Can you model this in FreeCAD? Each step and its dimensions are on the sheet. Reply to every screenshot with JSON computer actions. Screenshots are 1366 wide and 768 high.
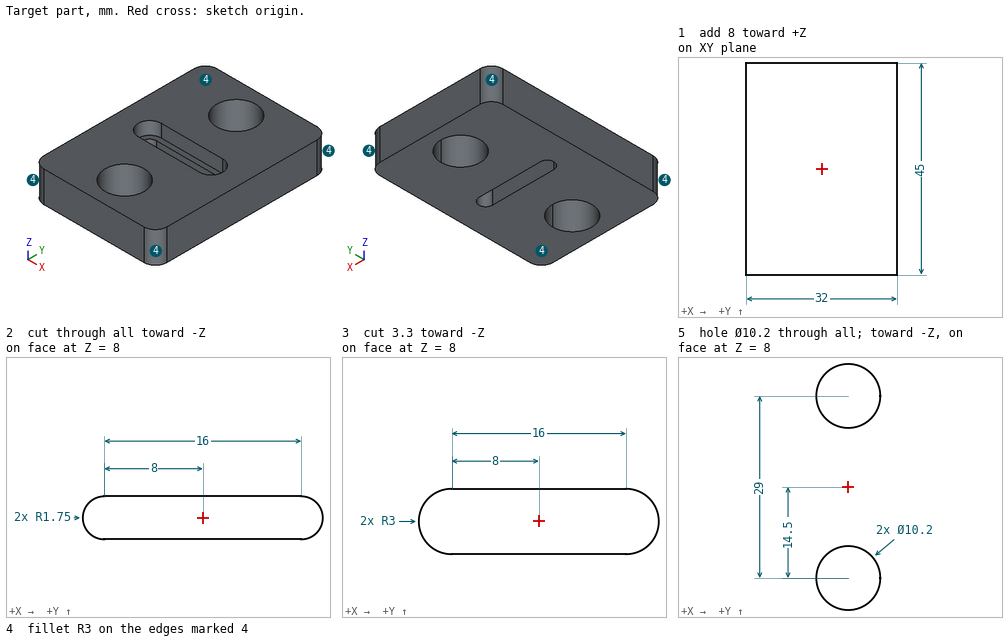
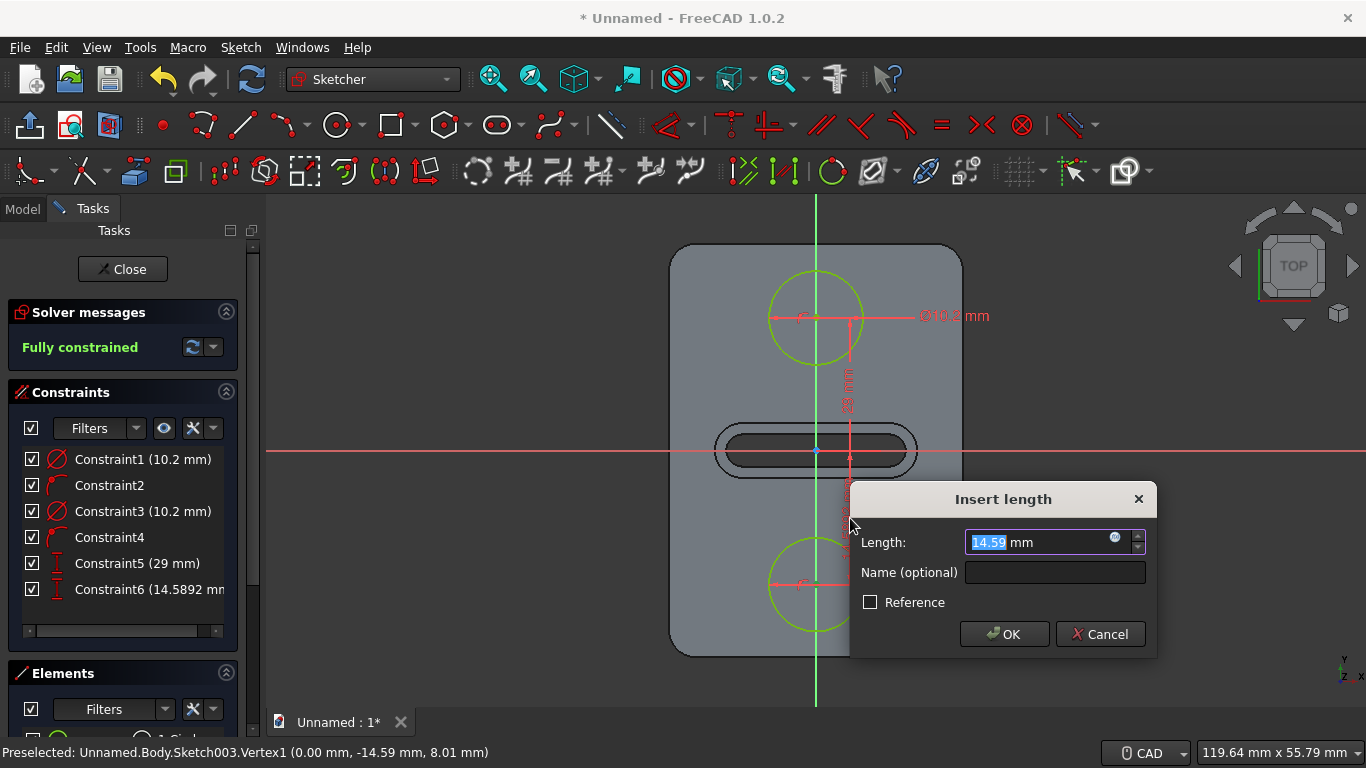
{"action": "type", "text": "14.5"}
{"action": "key", "text": "Return"}
{"action": "key", "text": "Escape"}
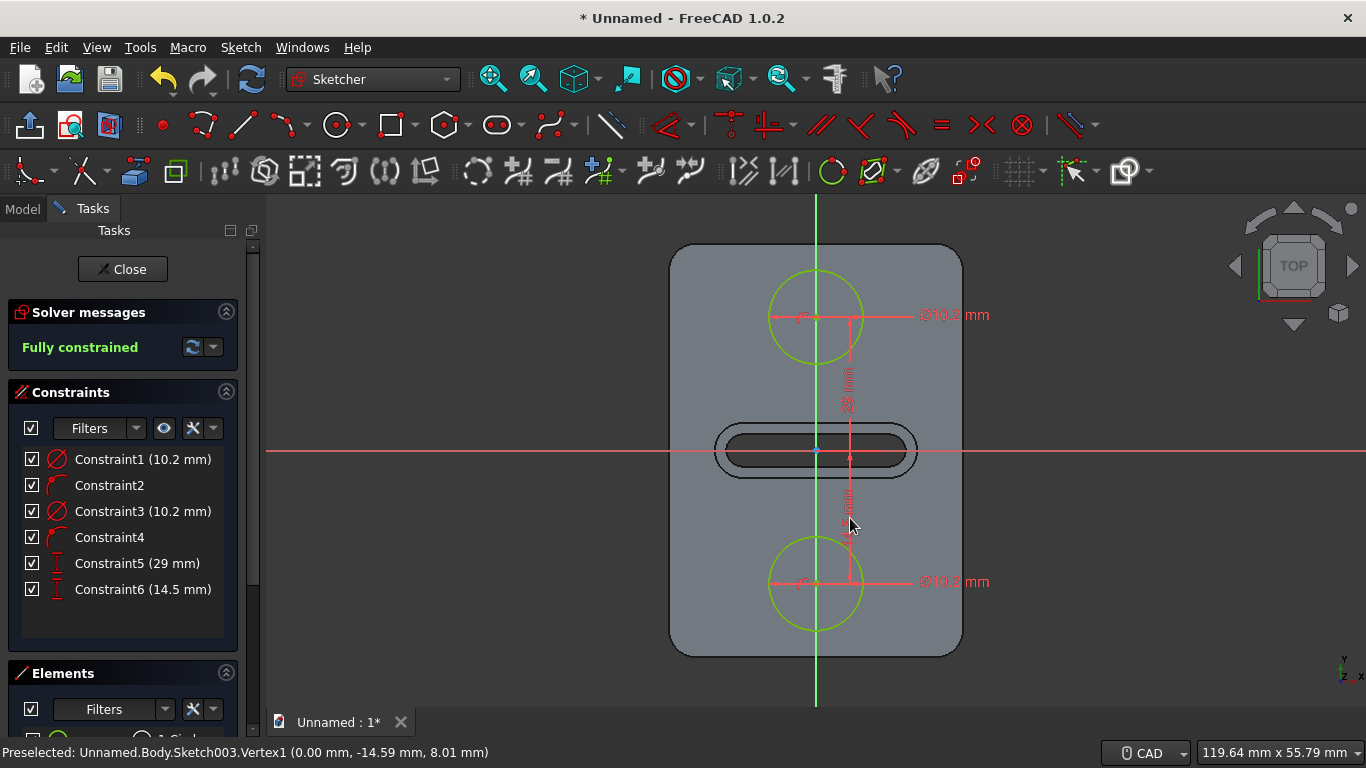
{"action": "left_click", "coordinate": [123, 269]}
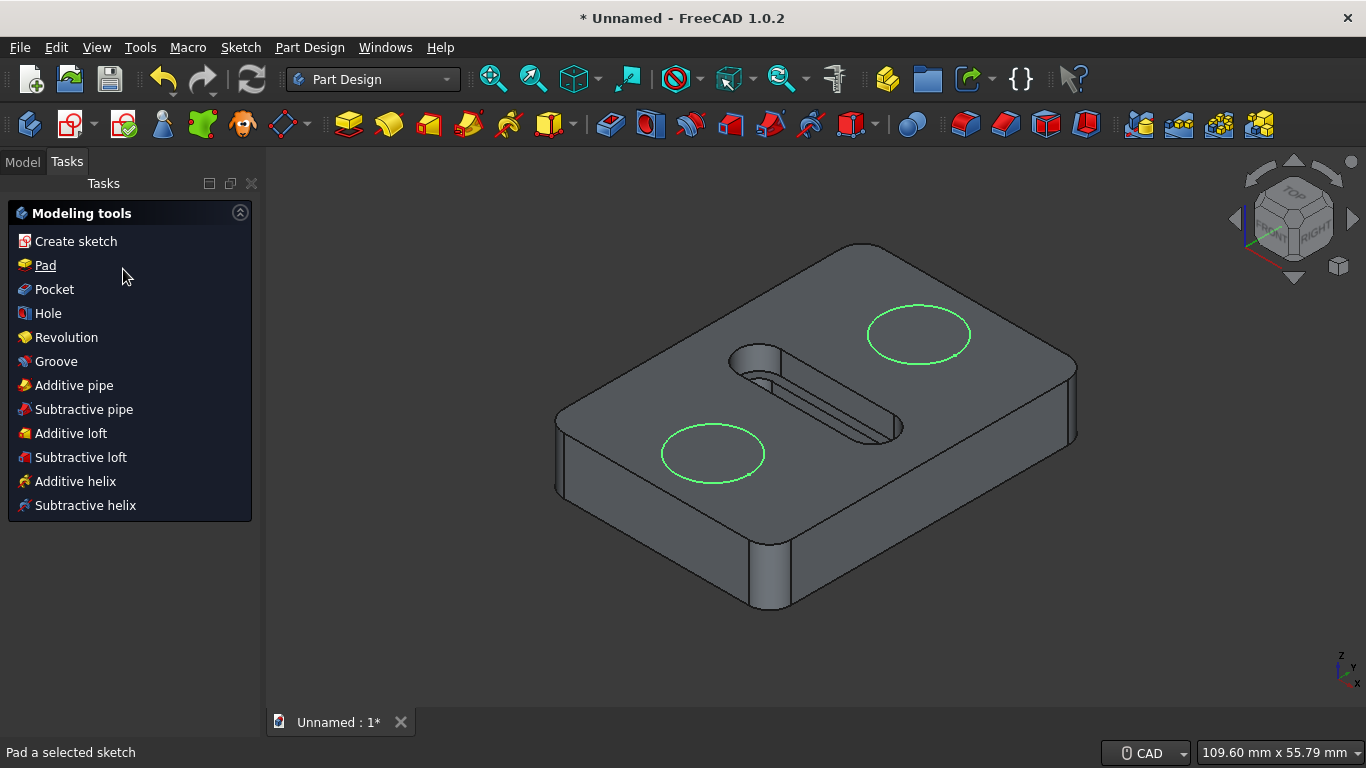
{"action": "left_click", "coordinate": [652, 124]}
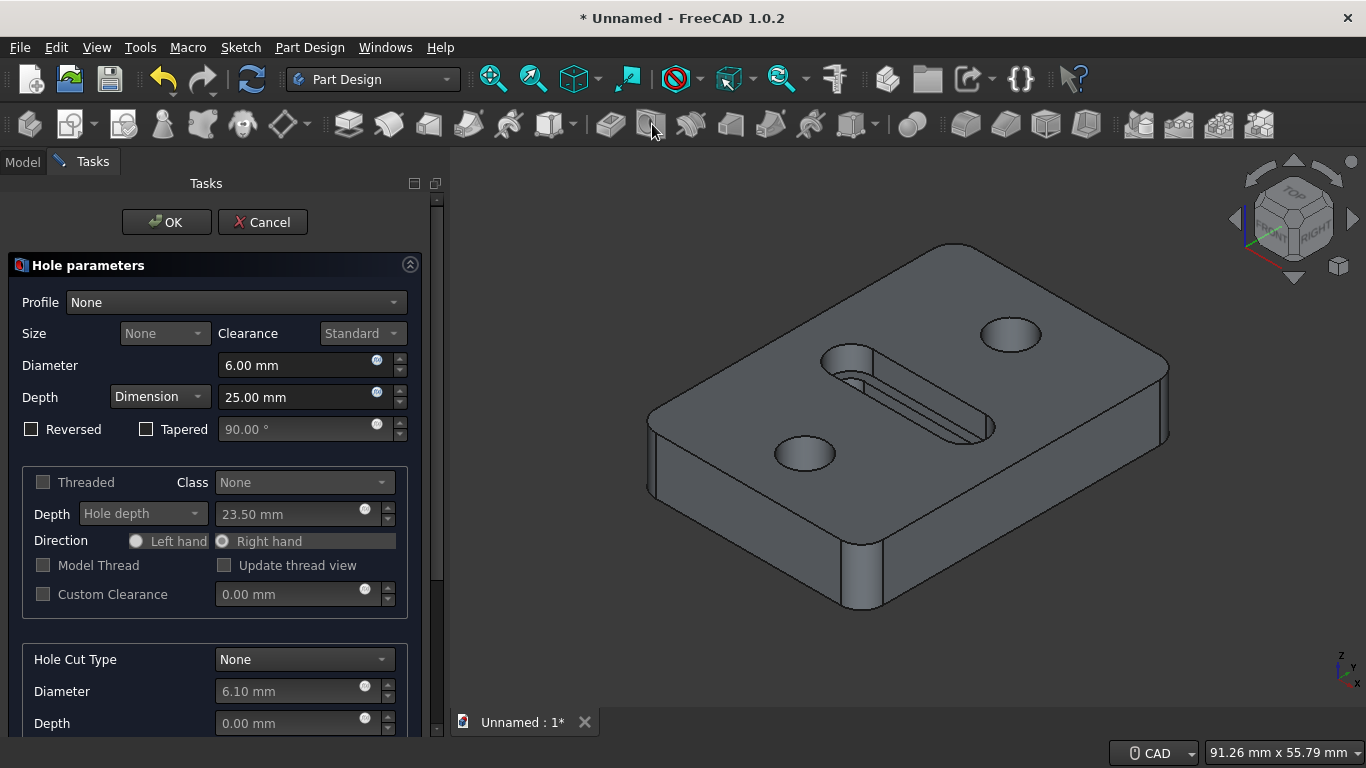
{"action": "triple_click", "coordinate": [305, 365]}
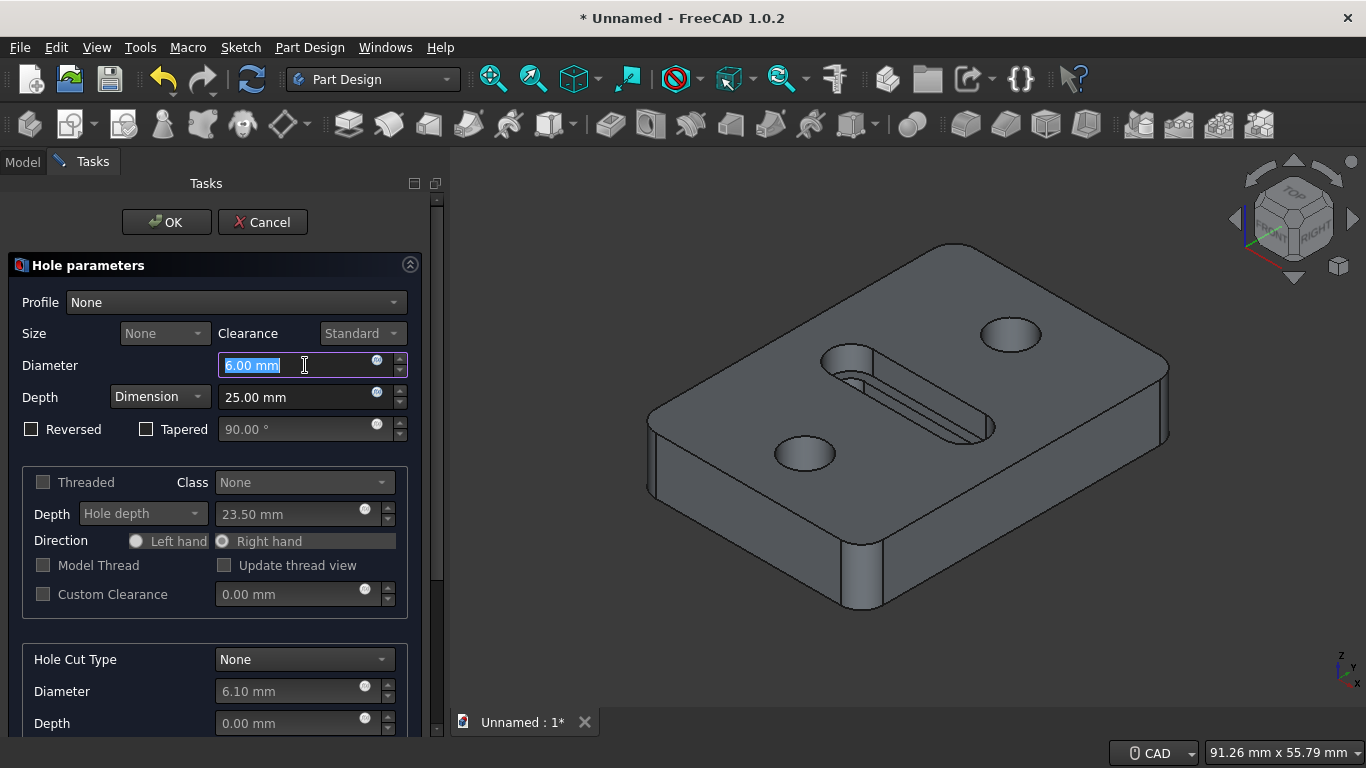
{"action": "type", "text": "10.2"}
{"action": "key", "text": "Tab"}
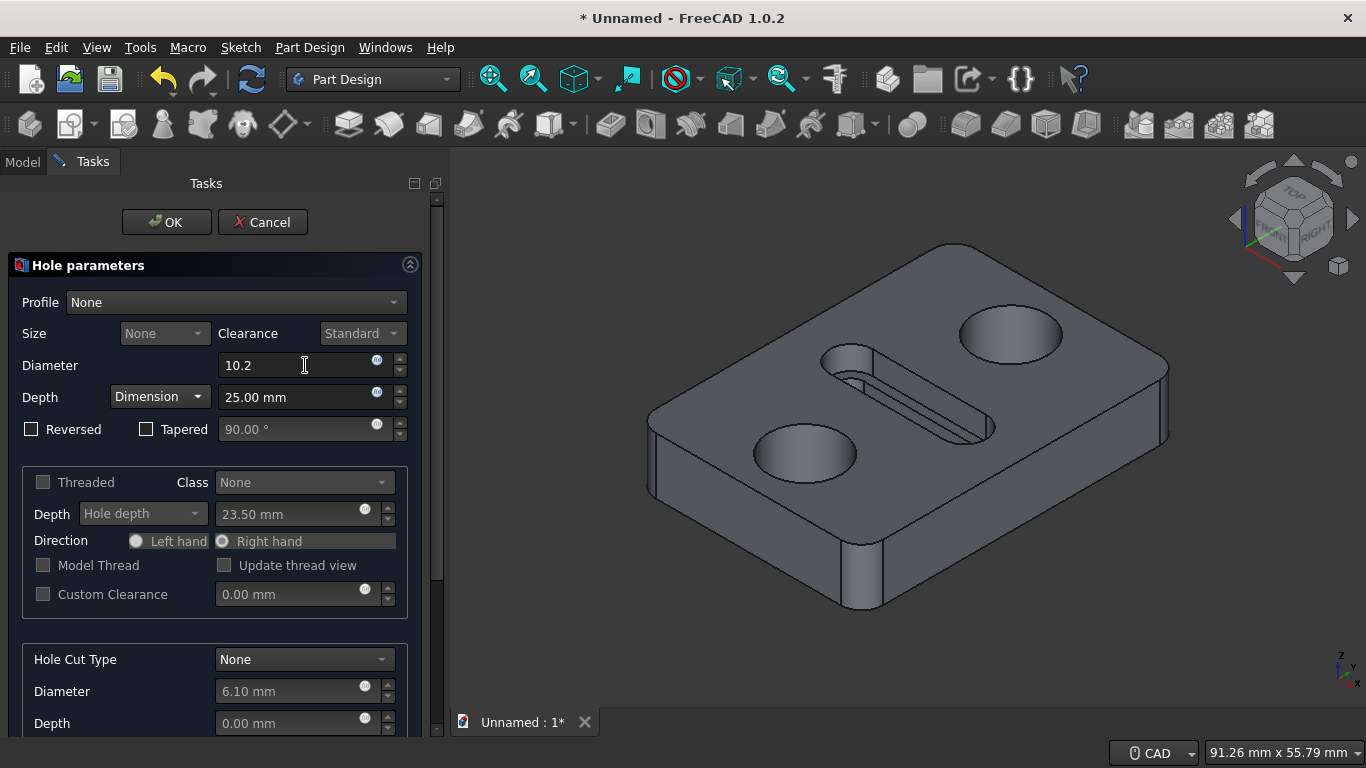
{"action": "left_click", "coordinate": [161, 396]}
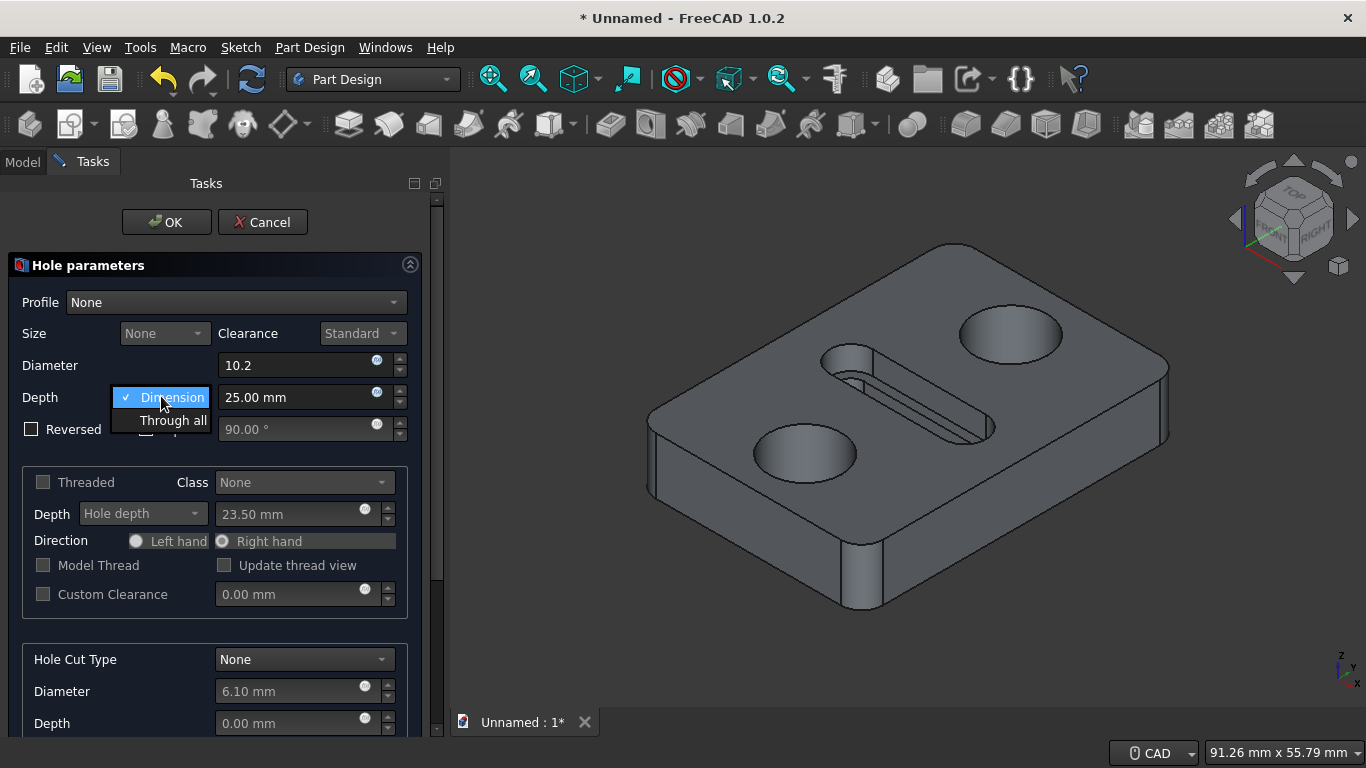
{"action": "left_click", "coordinate": [160, 420]}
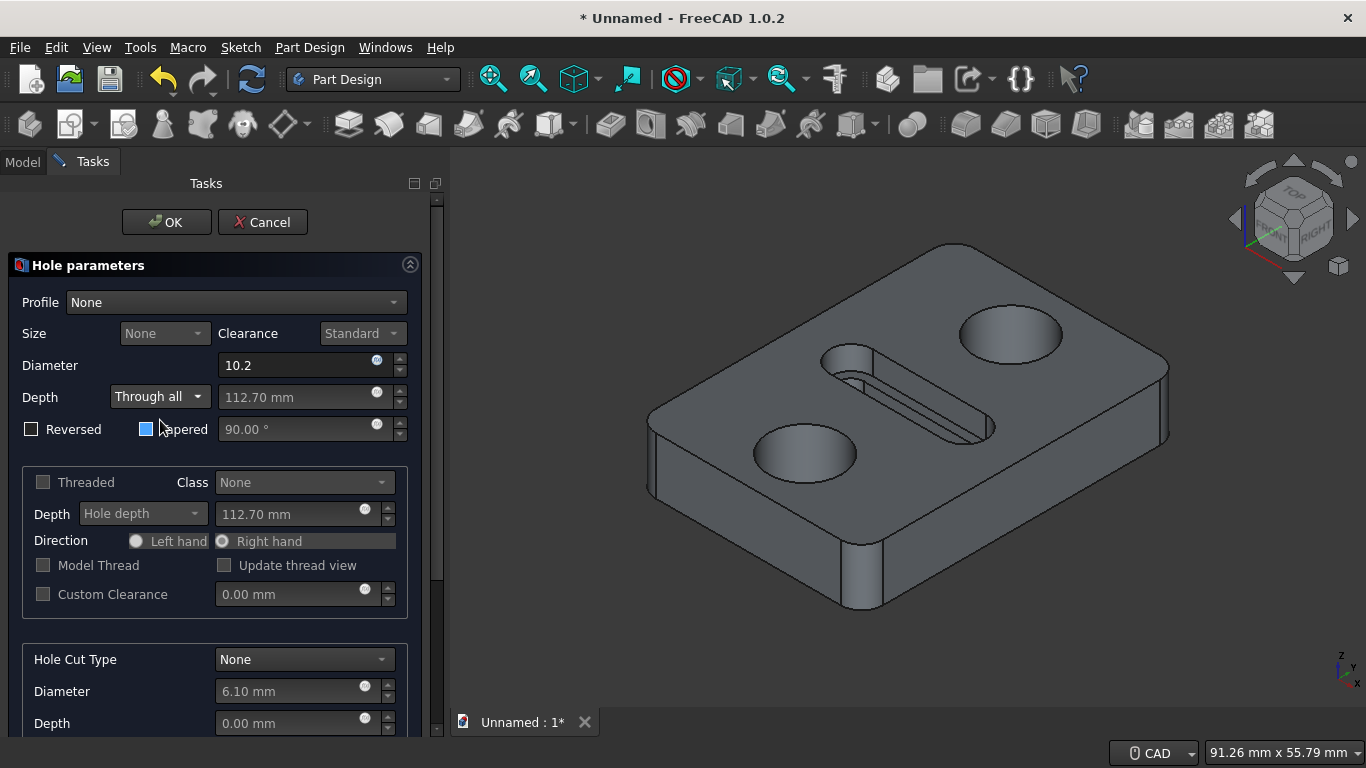
{"action": "left_click", "coordinate": [167, 222]}